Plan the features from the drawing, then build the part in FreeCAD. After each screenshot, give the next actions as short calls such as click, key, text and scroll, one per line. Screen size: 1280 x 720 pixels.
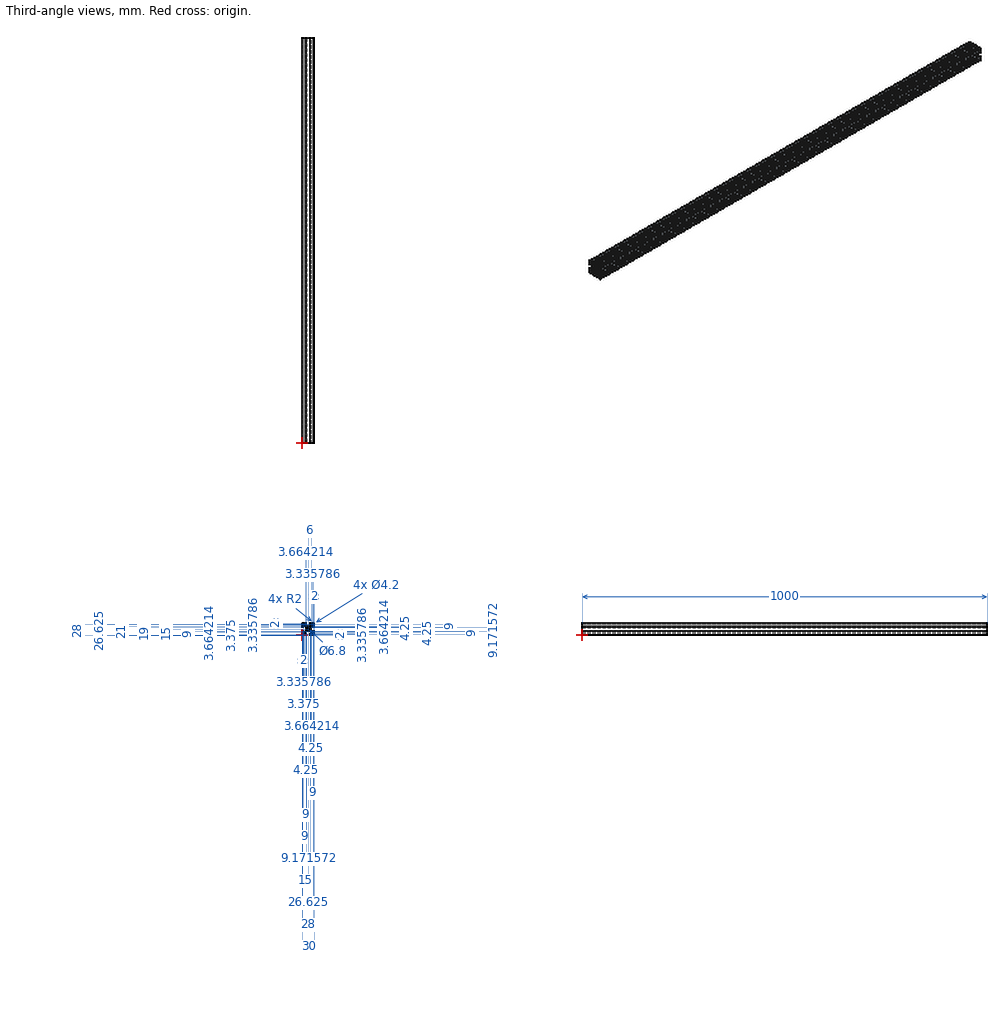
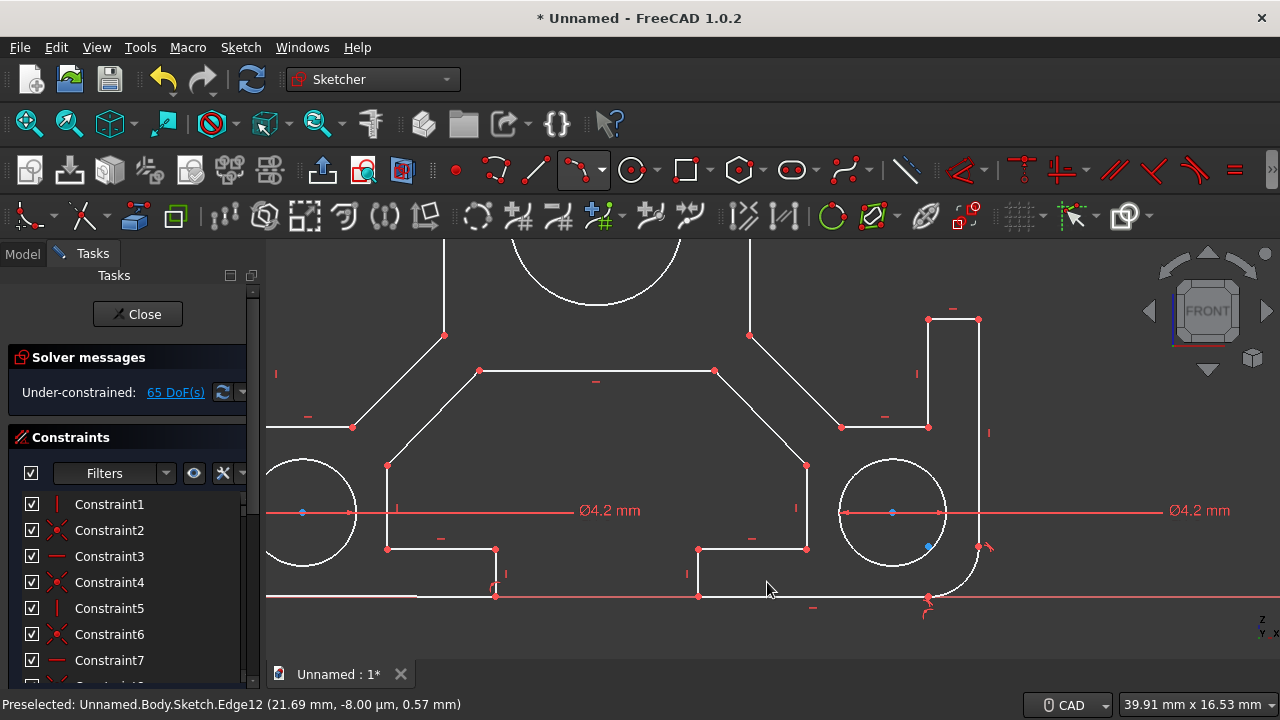
click(425, 597)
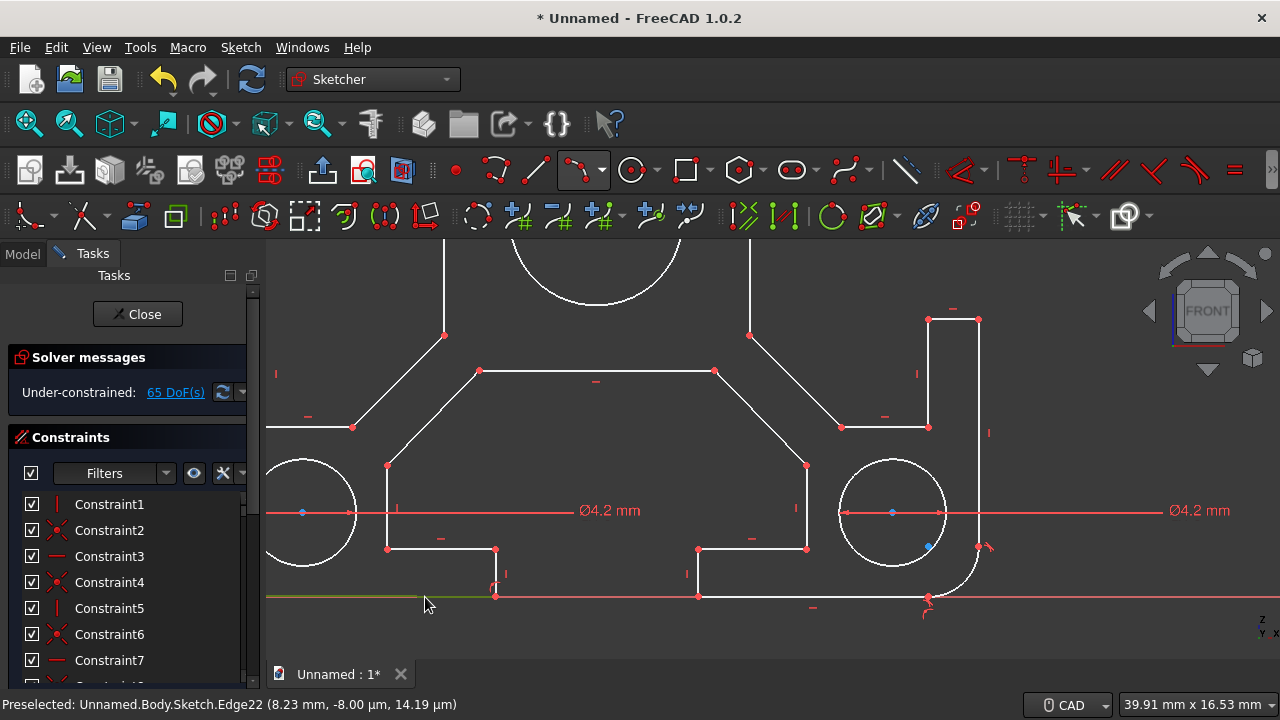
click(1088, 170)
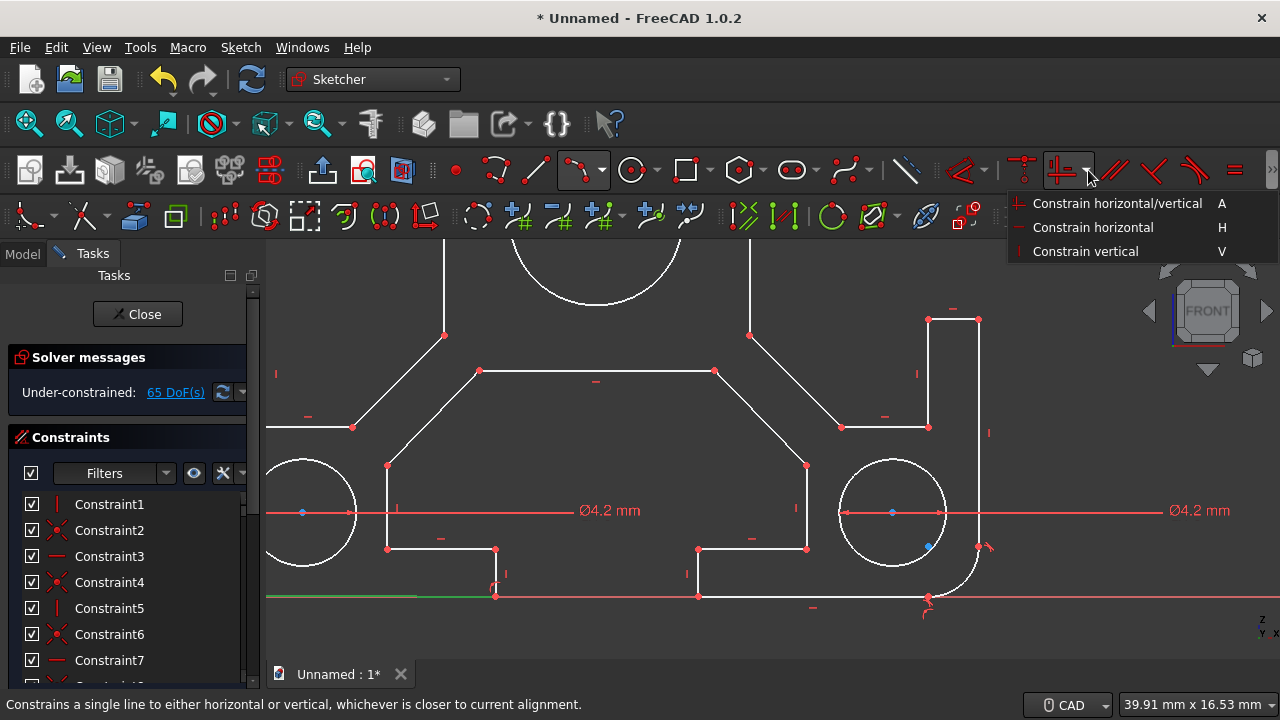
click(1143, 227)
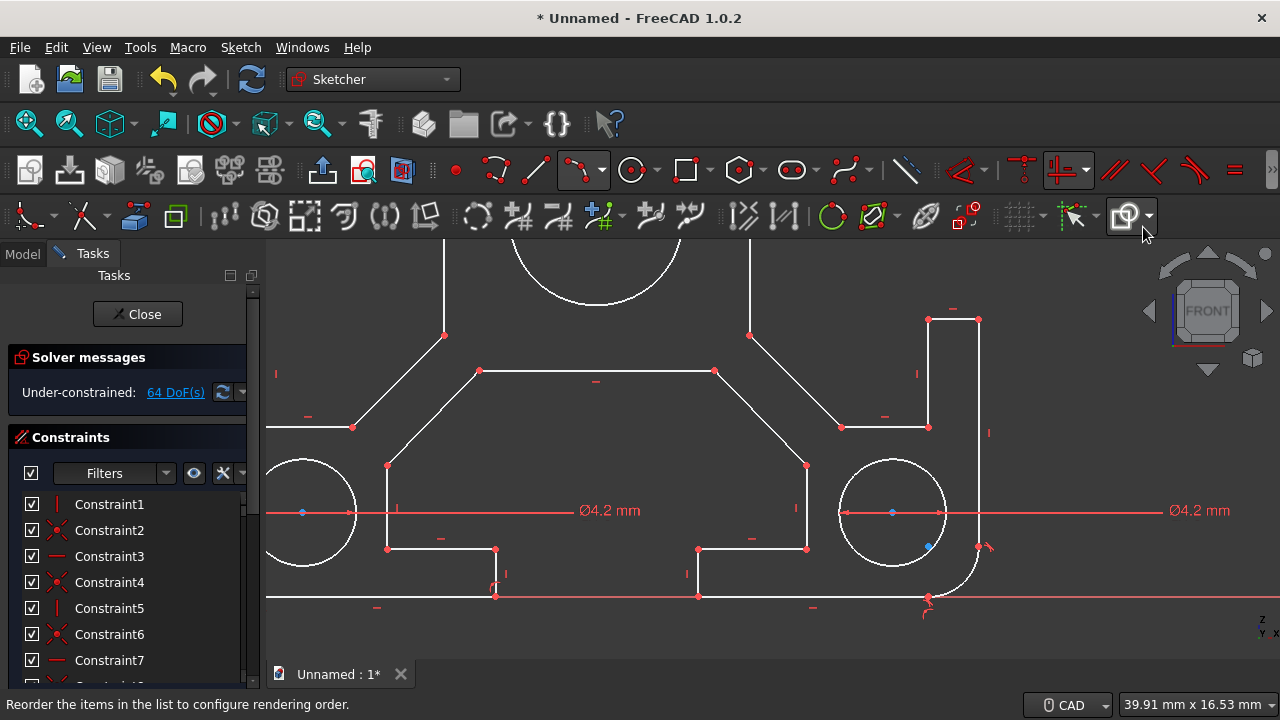
scroll(767, 585, down, 5)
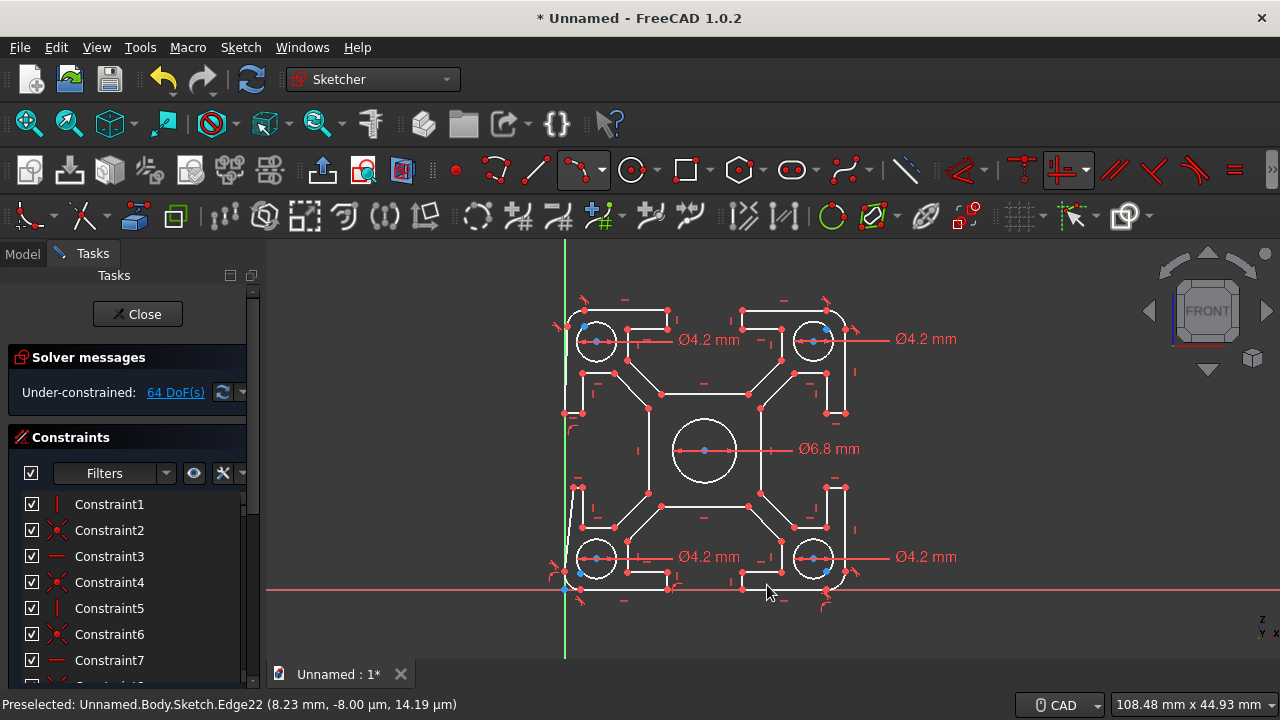
scroll(571, 513, up, 4)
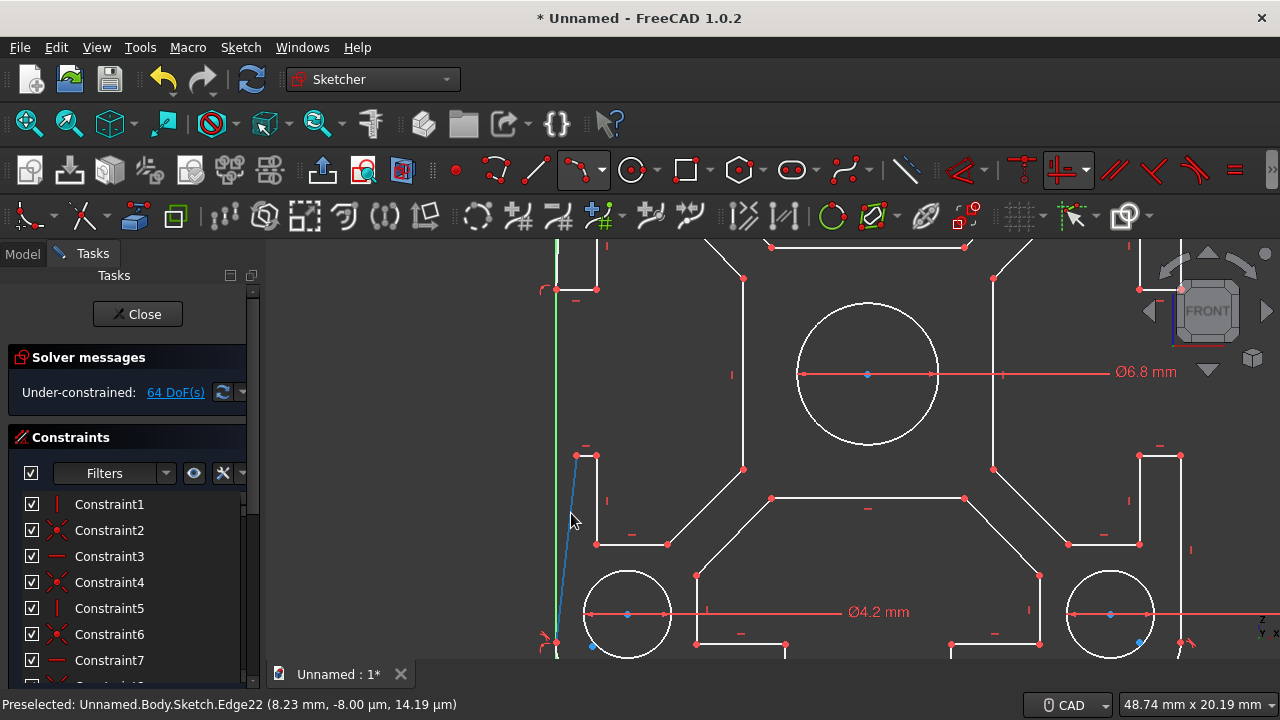
click(571, 512)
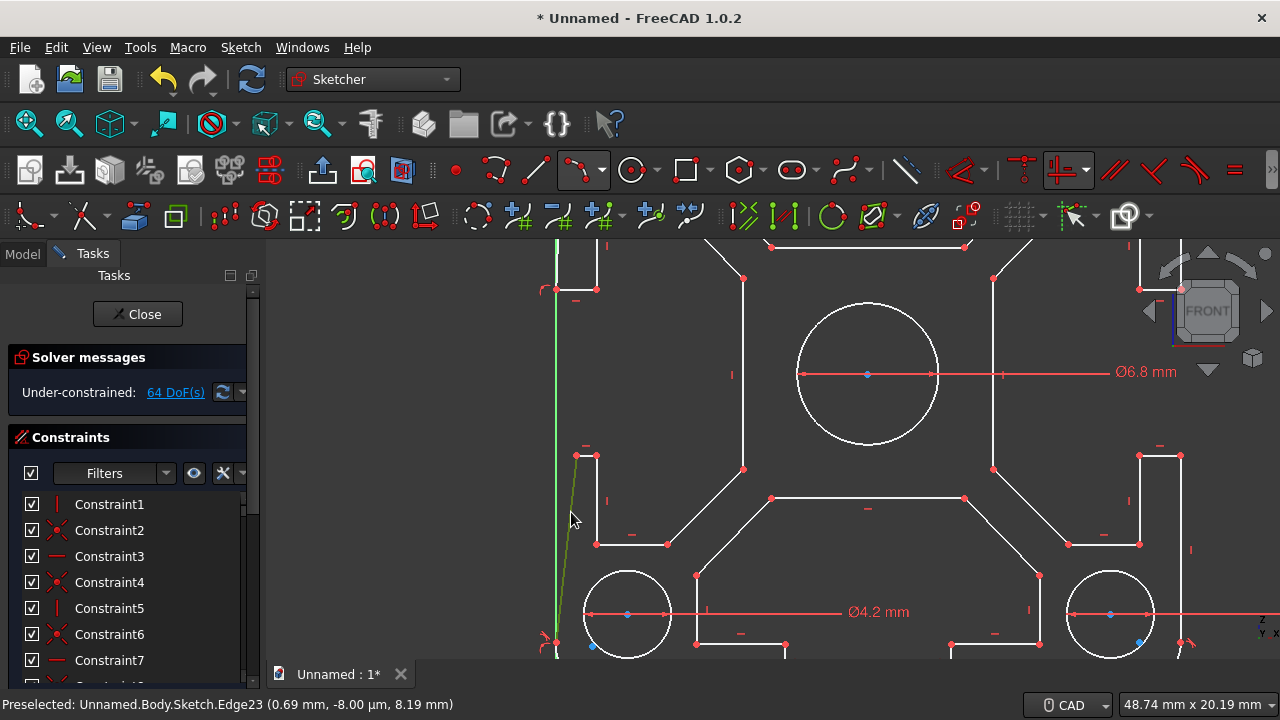
key(v)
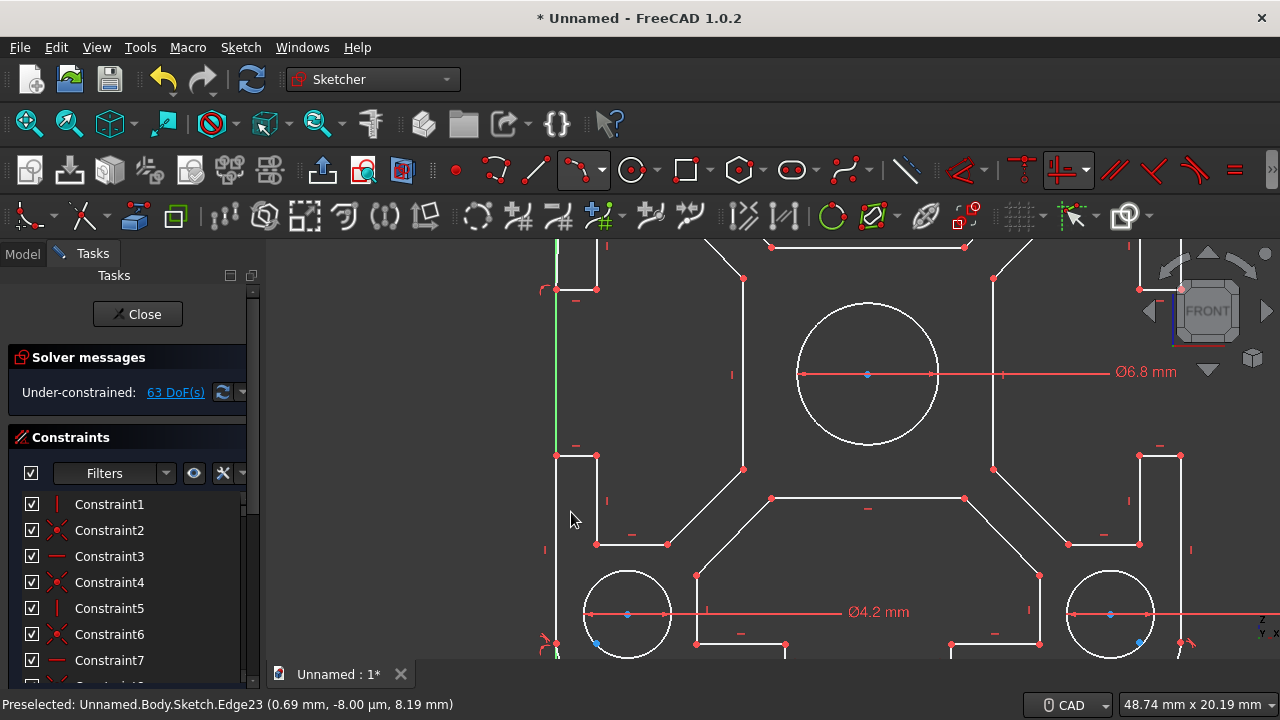
scroll(571, 512, down, 4)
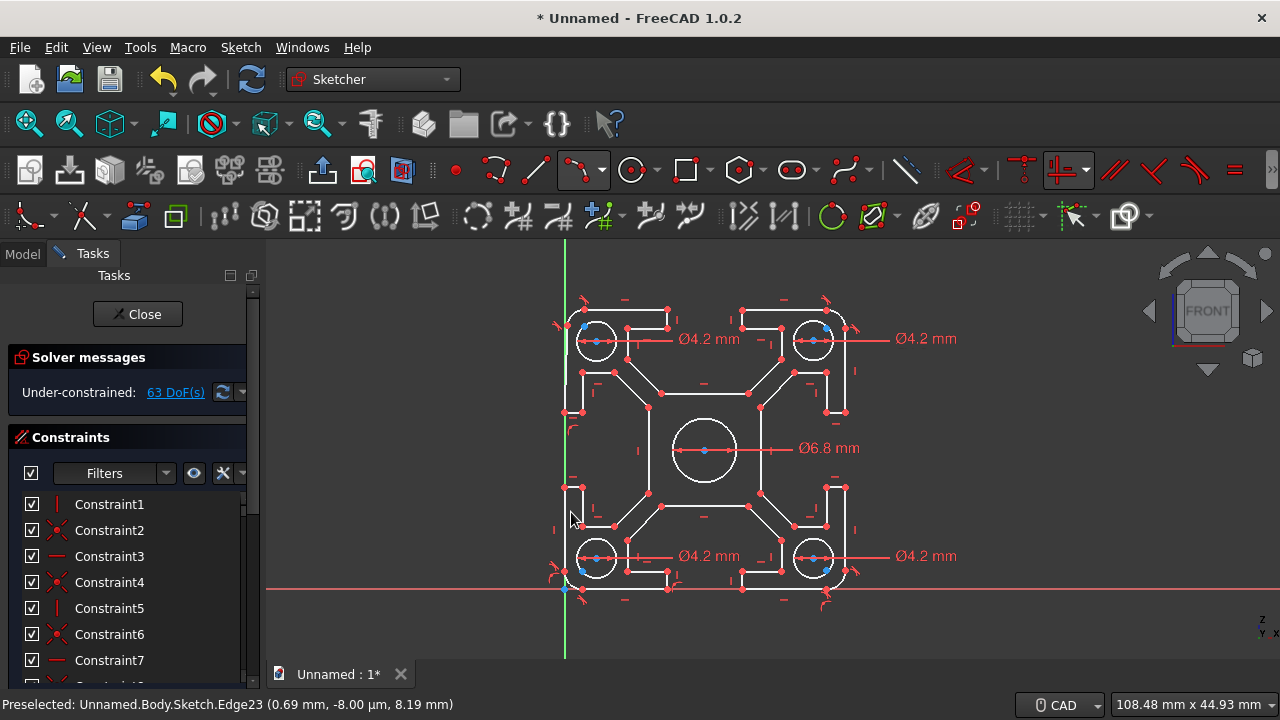
click(565, 387)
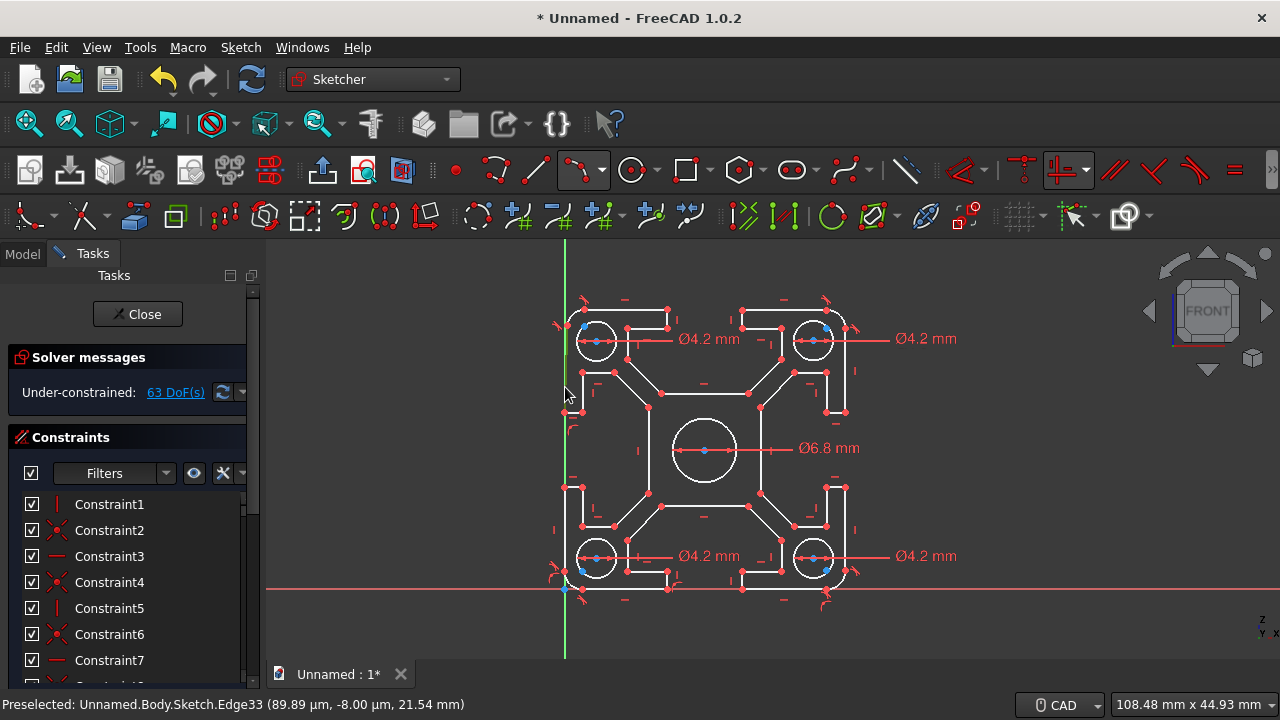
key(v)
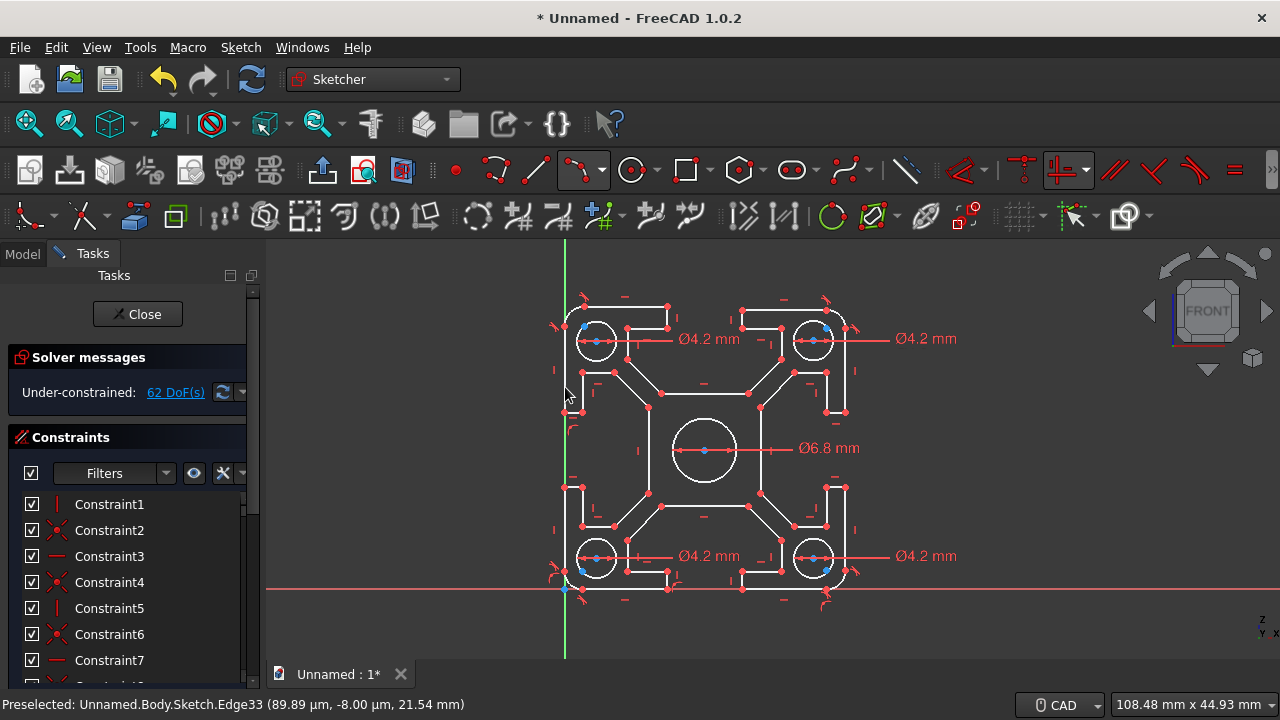
scroll(843, 579, up, 3)